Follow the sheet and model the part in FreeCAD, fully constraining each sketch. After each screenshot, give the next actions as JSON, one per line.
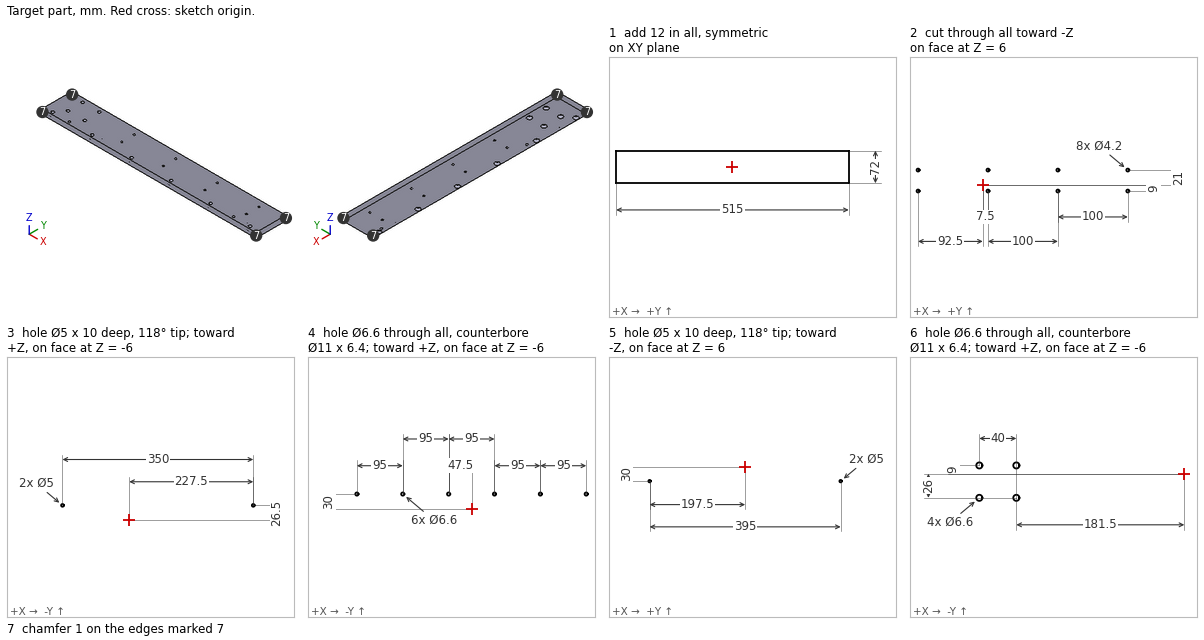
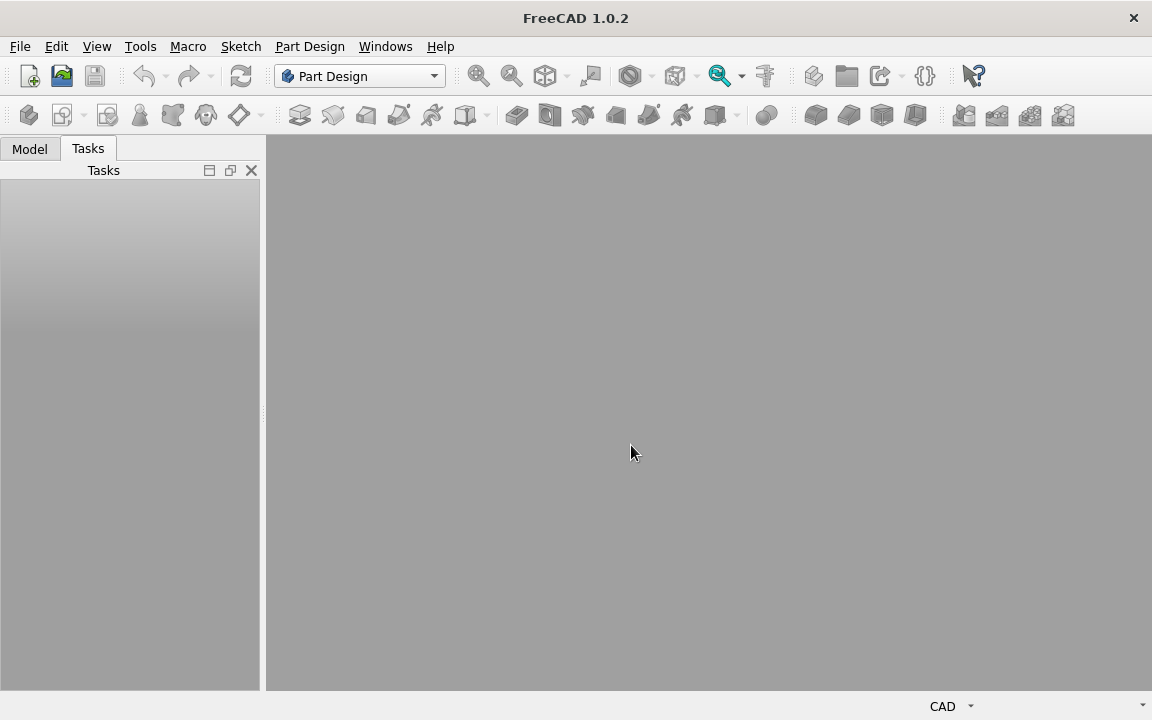
{"action": "left_click", "coordinate": [29, 76]}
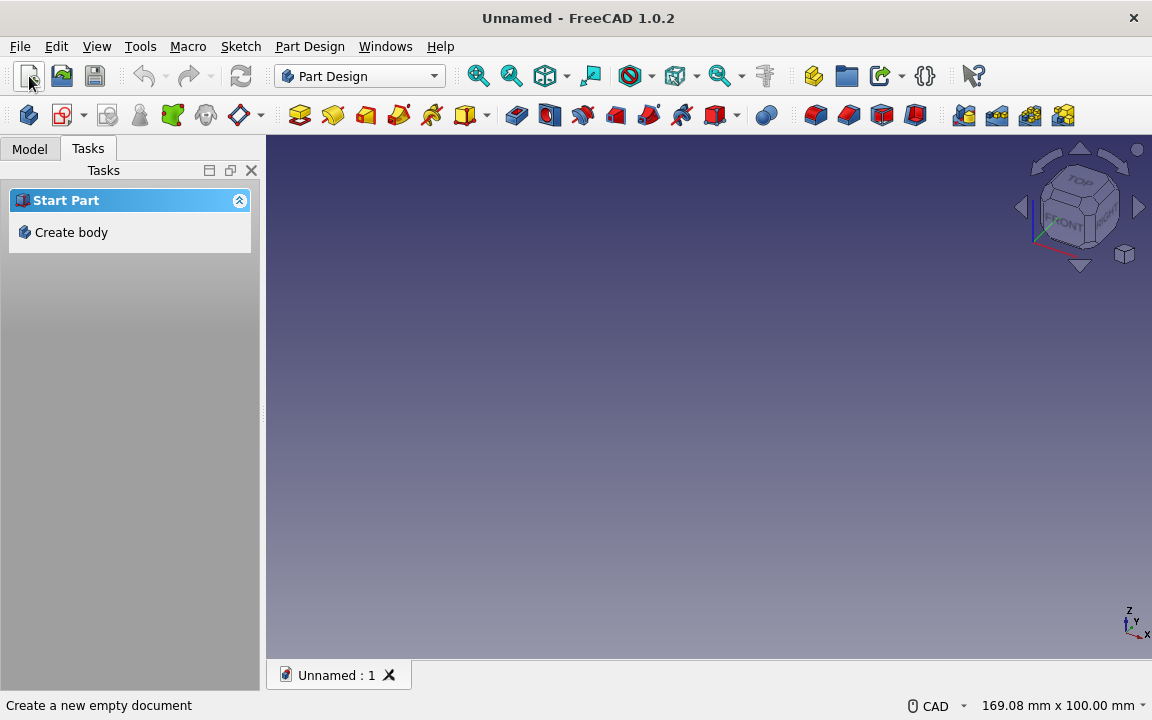
{"action": "left_click", "coordinate": [62, 116]}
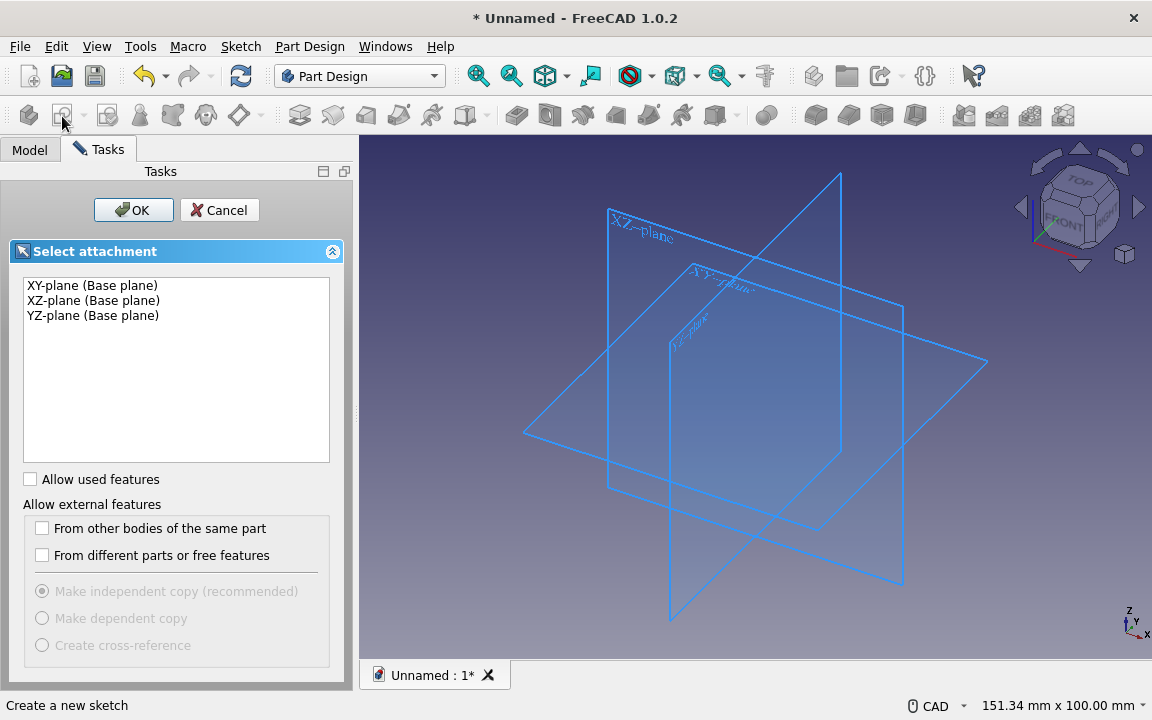
{"action": "left_click", "coordinate": [84, 286]}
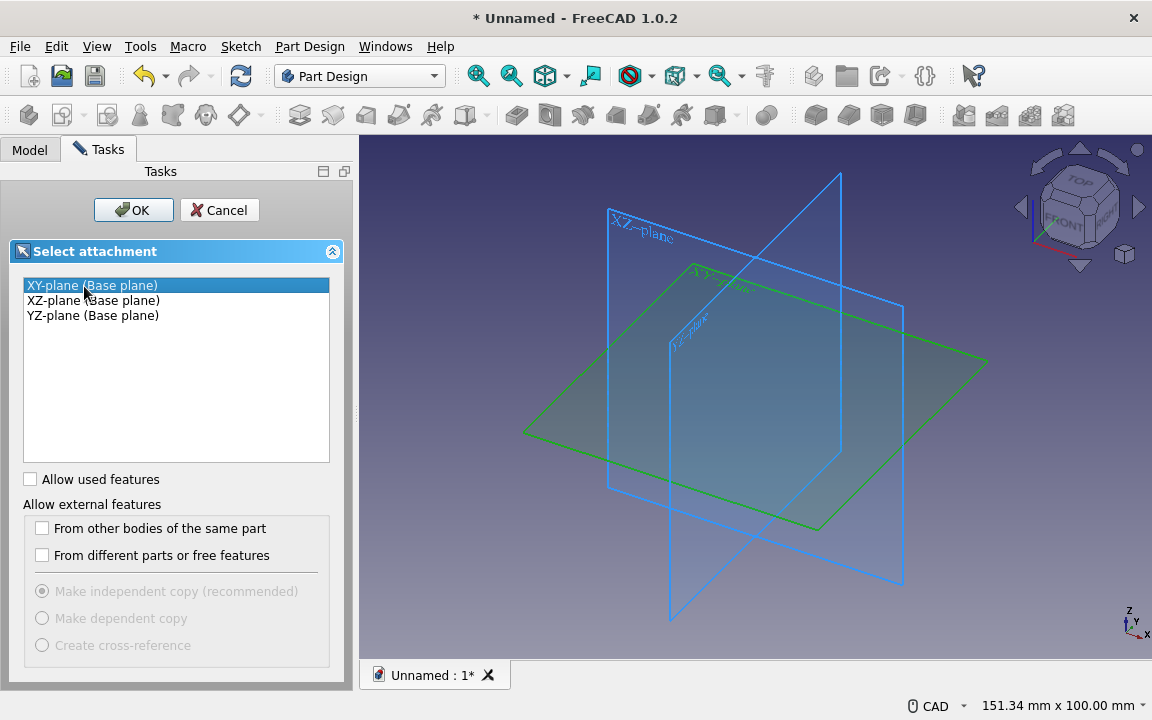
{"action": "left_click", "coordinate": [134, 210]}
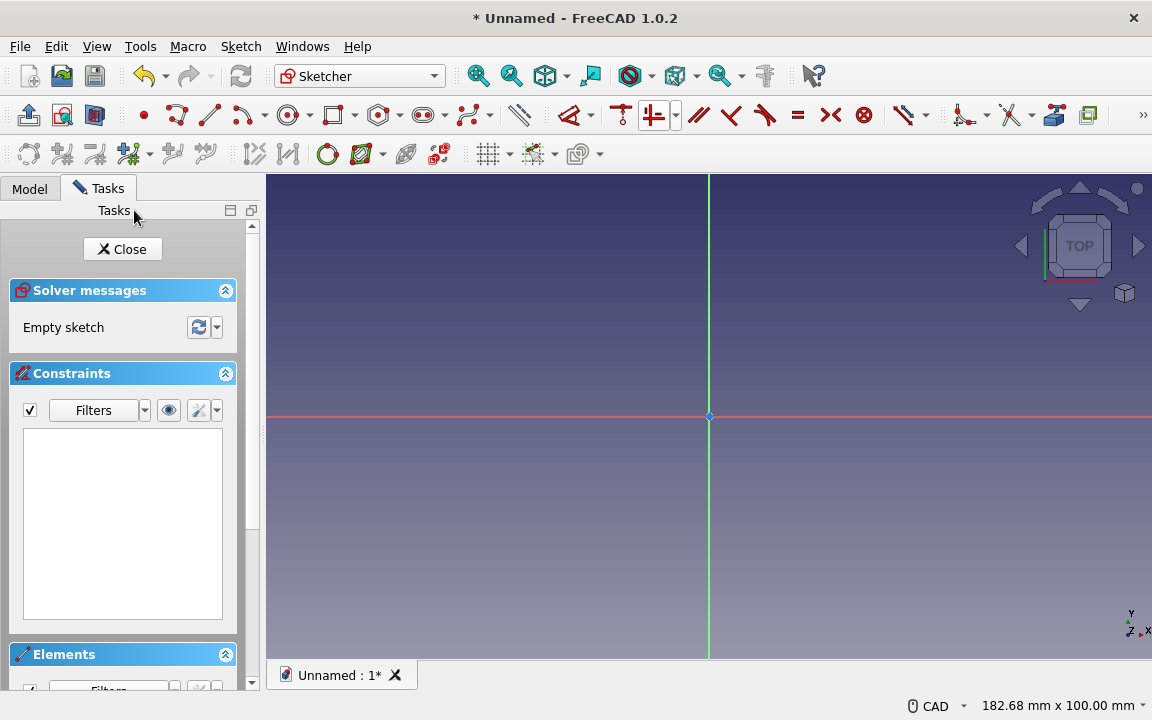
{"action": "scroll", "coordinate": [623, 416], "scroll_direction": "down", "scroll_amount": 8}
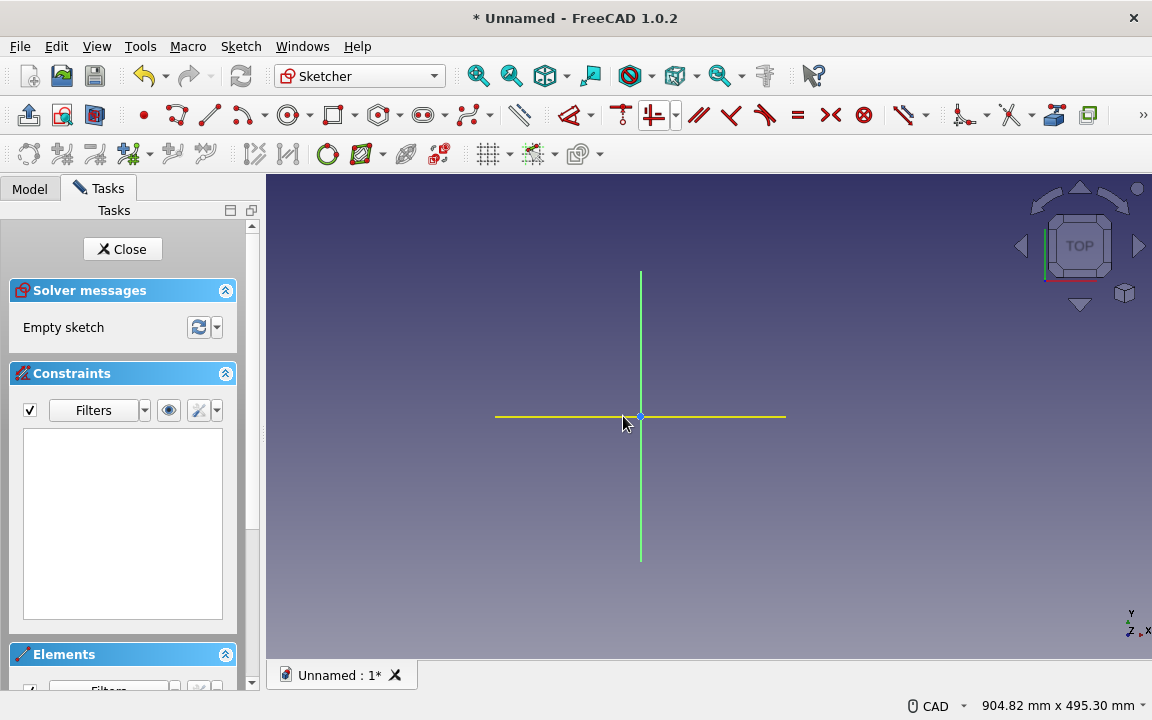
{"action": "key", "text": "g v"}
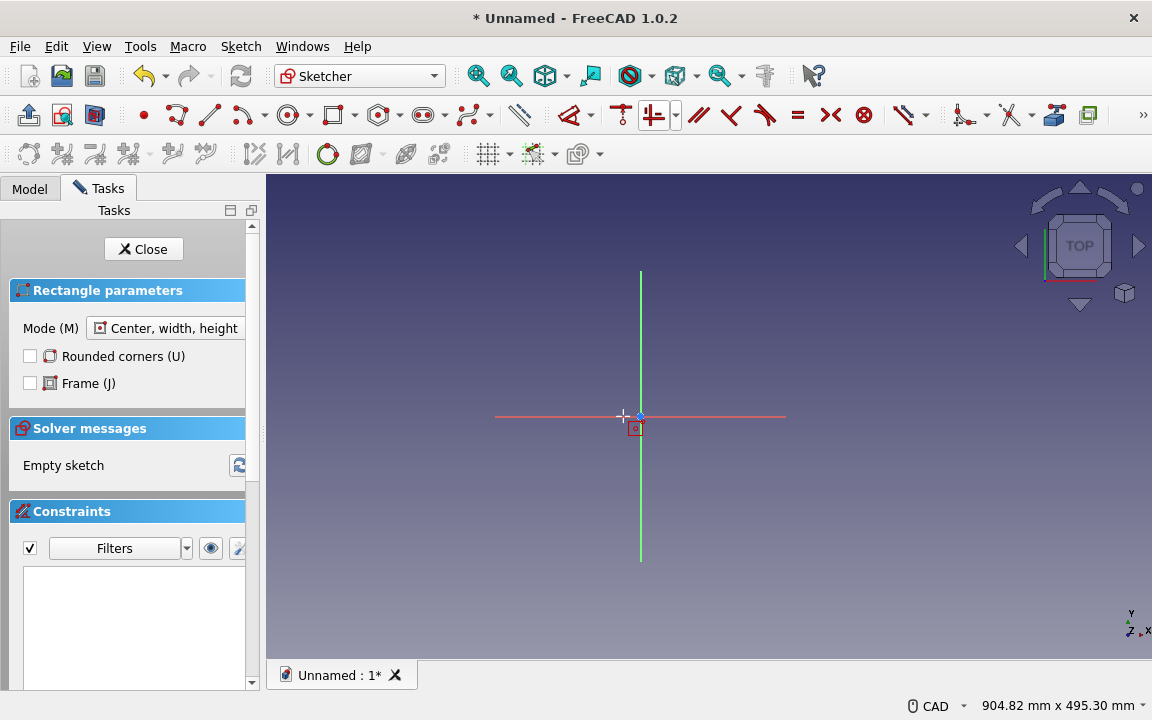
{"action": "left_click", "coordinate": [641, 416]}
{"action": "mouse_move", "coordinate": [893, 381]}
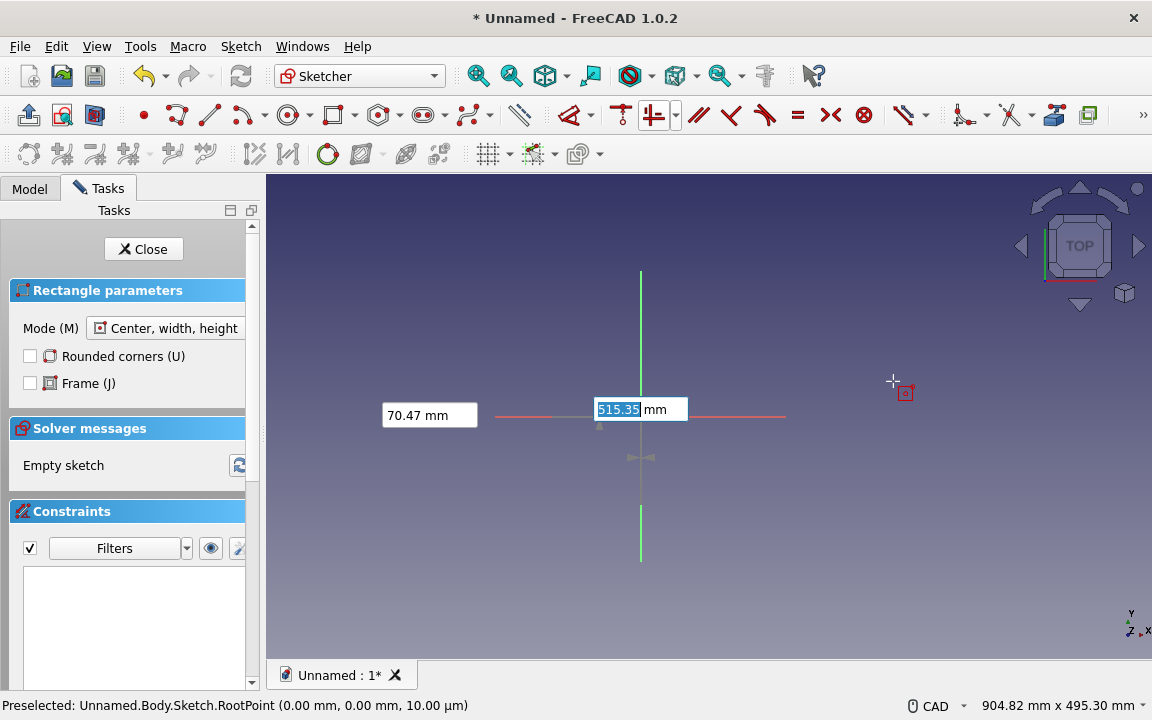
{"action": "type", "text": "515"}
{"action": "key", "text": "Tab"}
{"action": "type", "text": "72"}
{"action": "key", "text": "Return"}
{"action": "key", "text": "Escape"}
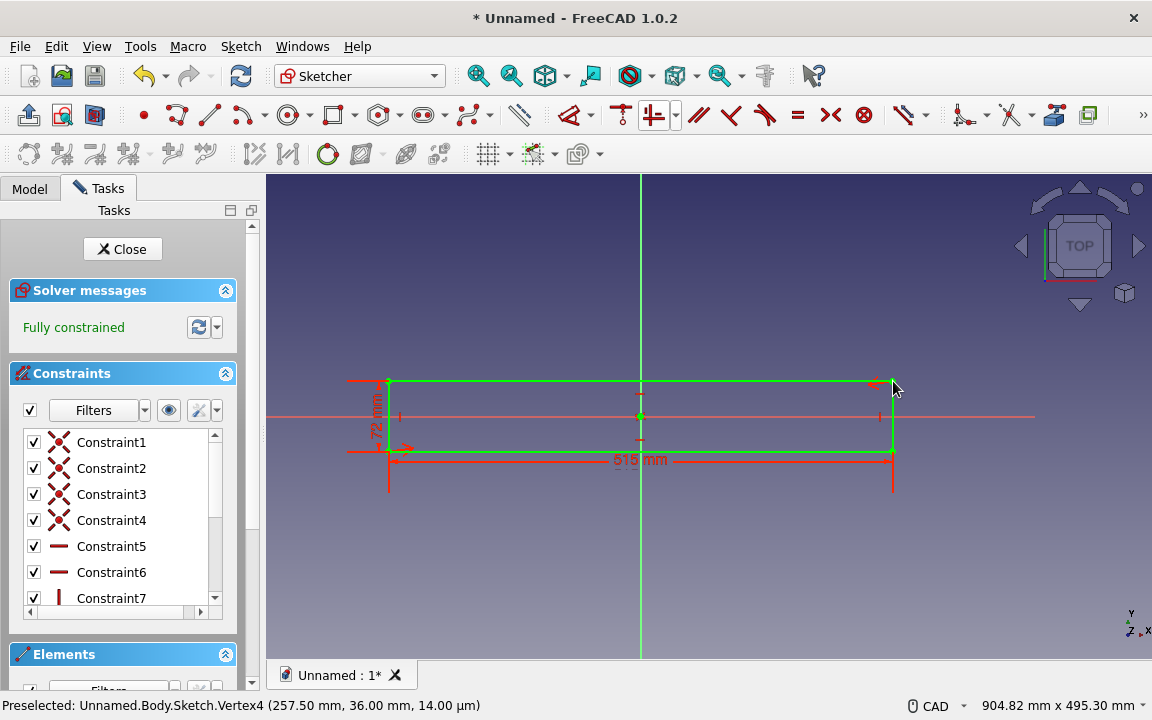
{"action": "left_click", "coordinate": [123, 249]}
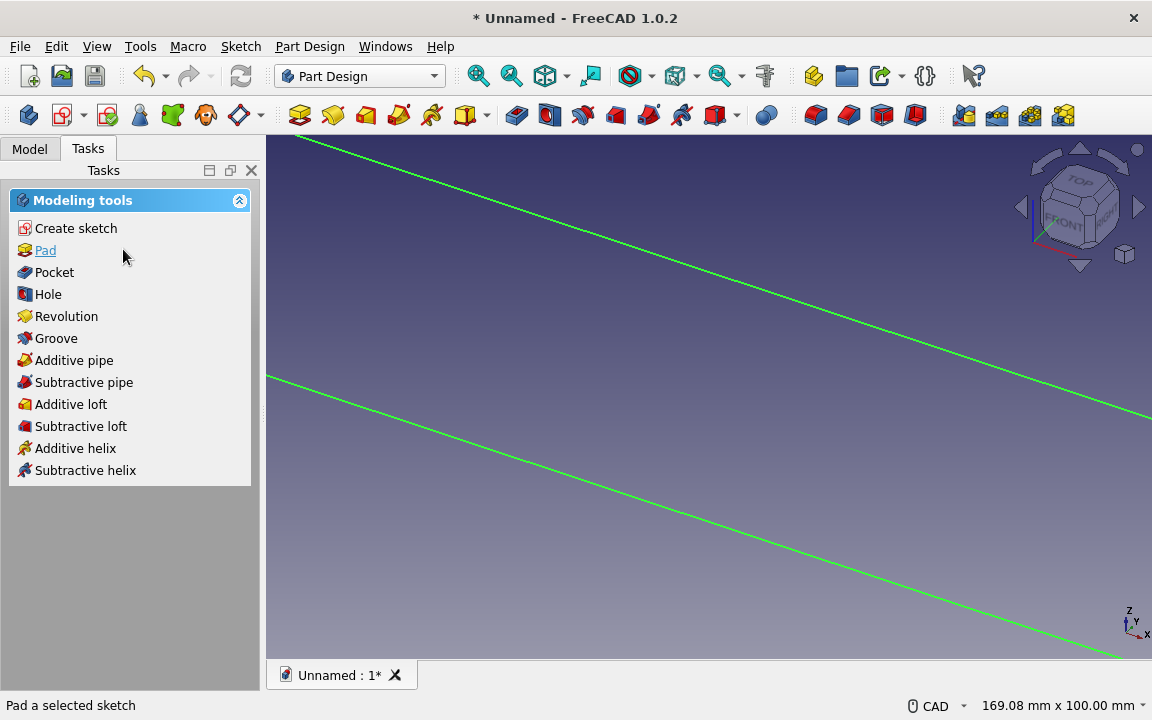
{"action": "left_click", "coordinate": [300, 116]}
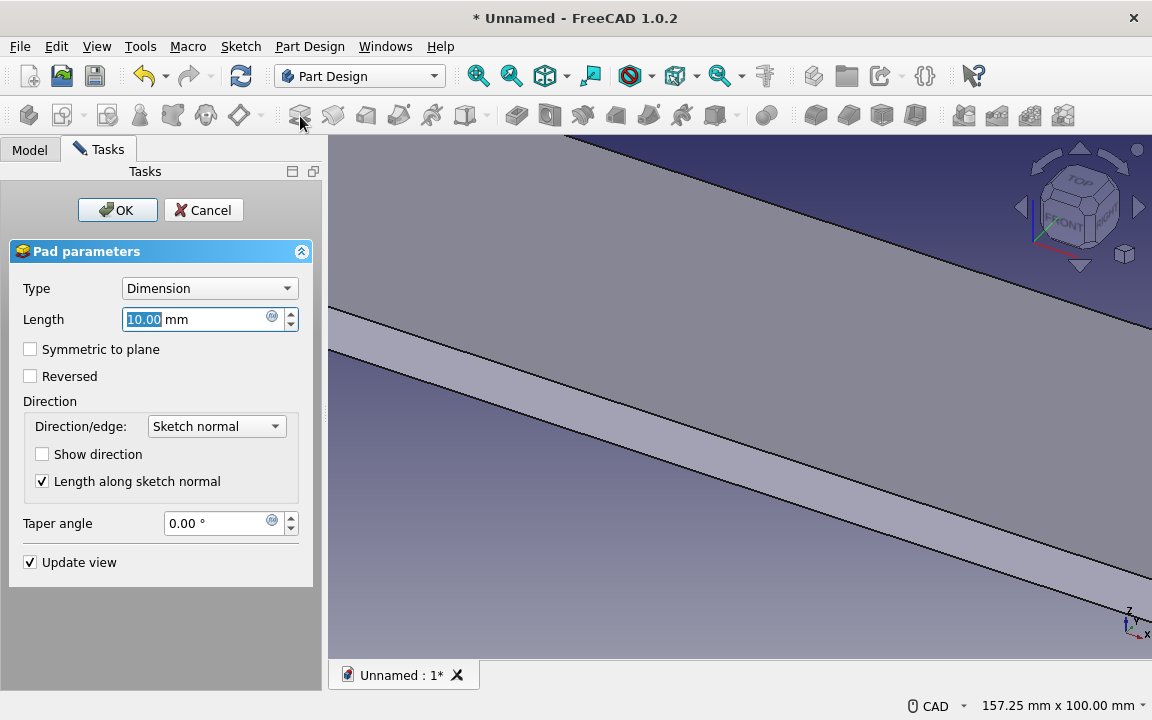
{"action": "type", "text": "12"}
{"action": "key", "text": "Tab"}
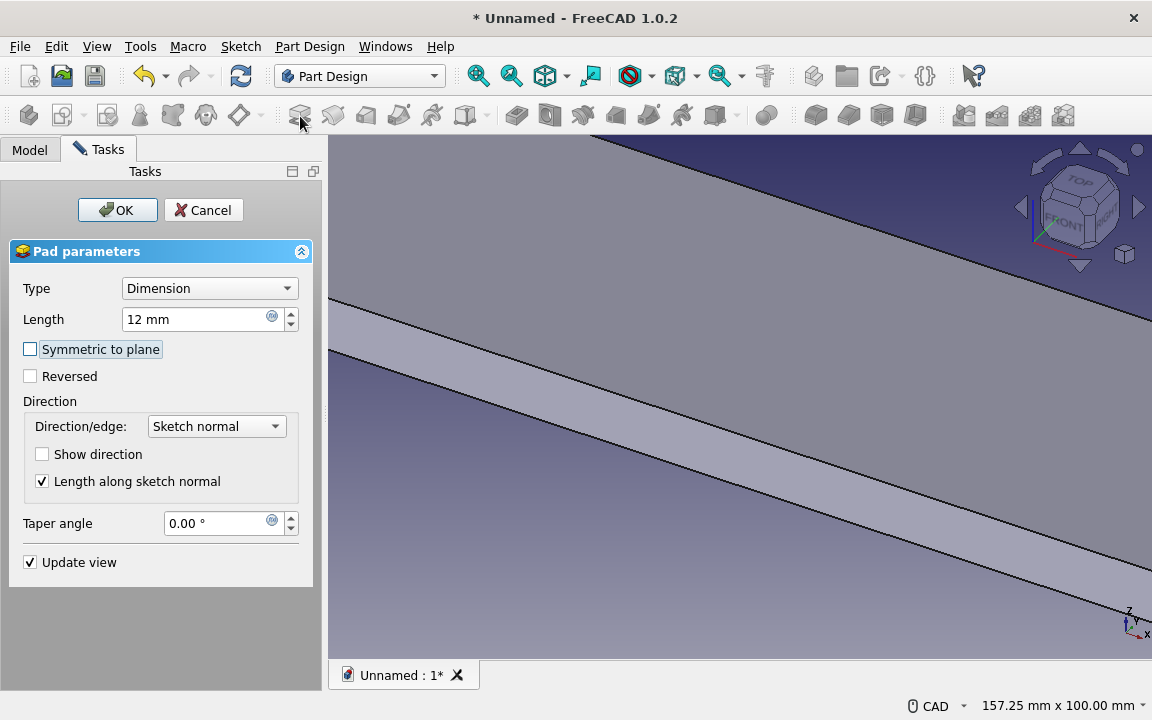
{"action": "left_click", "coordinate": [31, 349]}